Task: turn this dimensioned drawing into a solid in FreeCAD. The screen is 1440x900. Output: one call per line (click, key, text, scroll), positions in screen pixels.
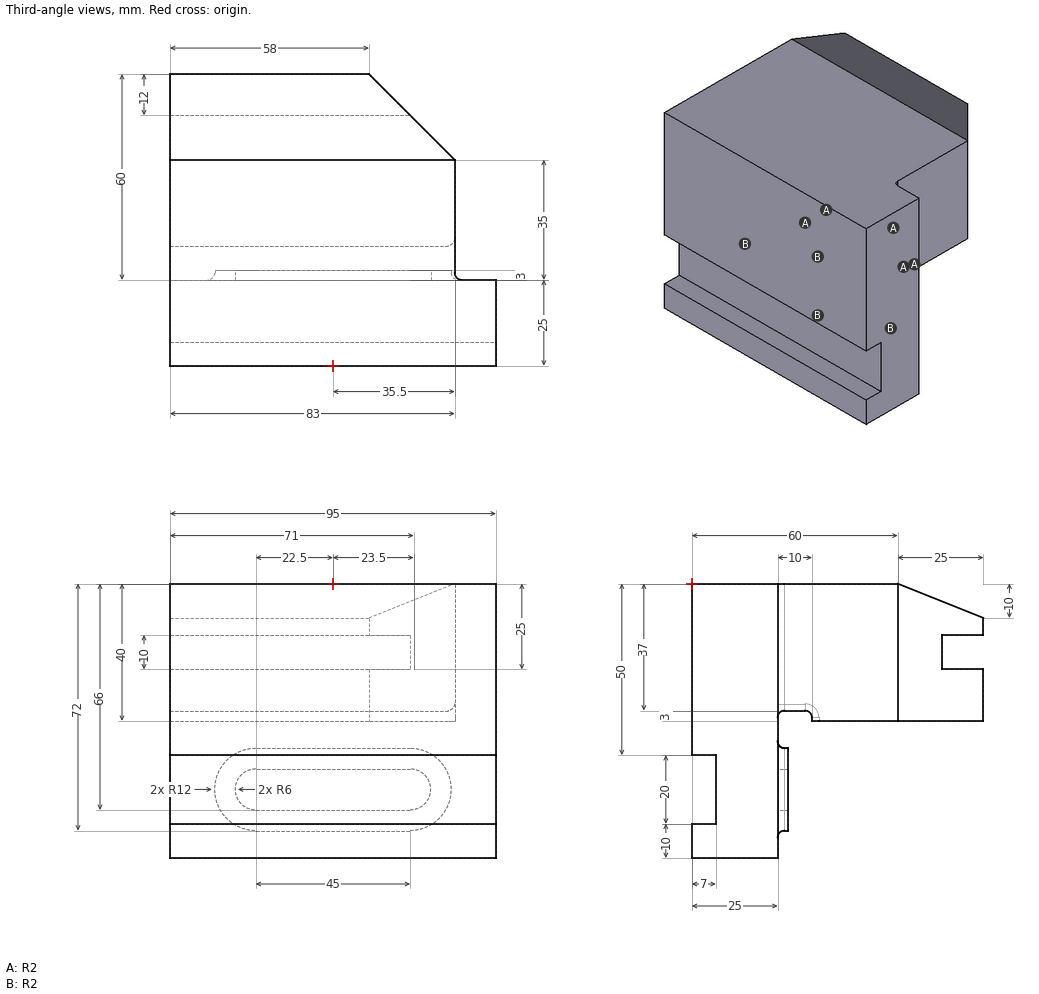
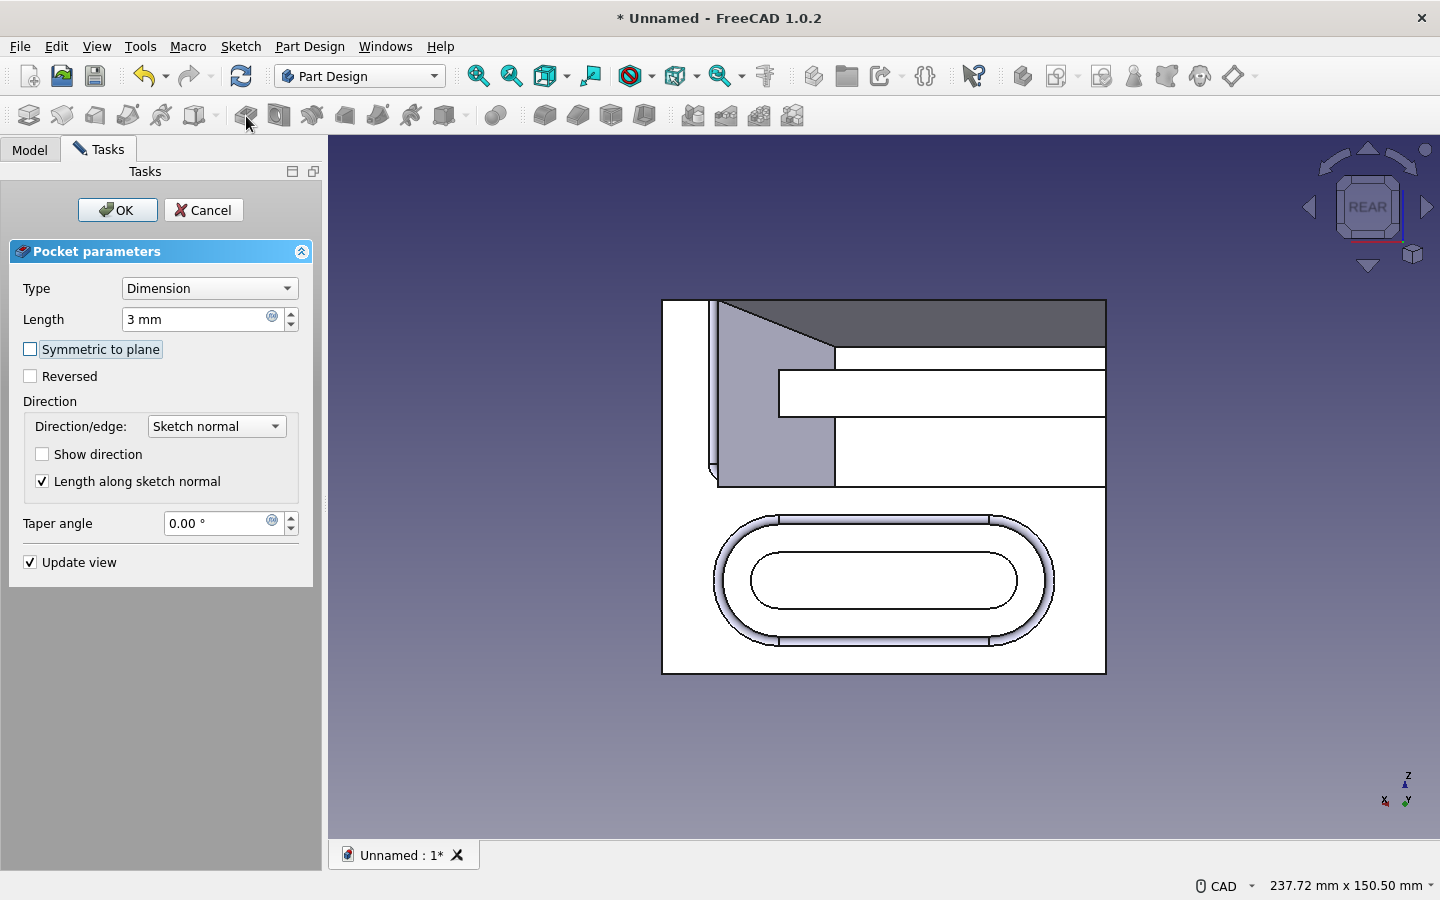
click(118, 210)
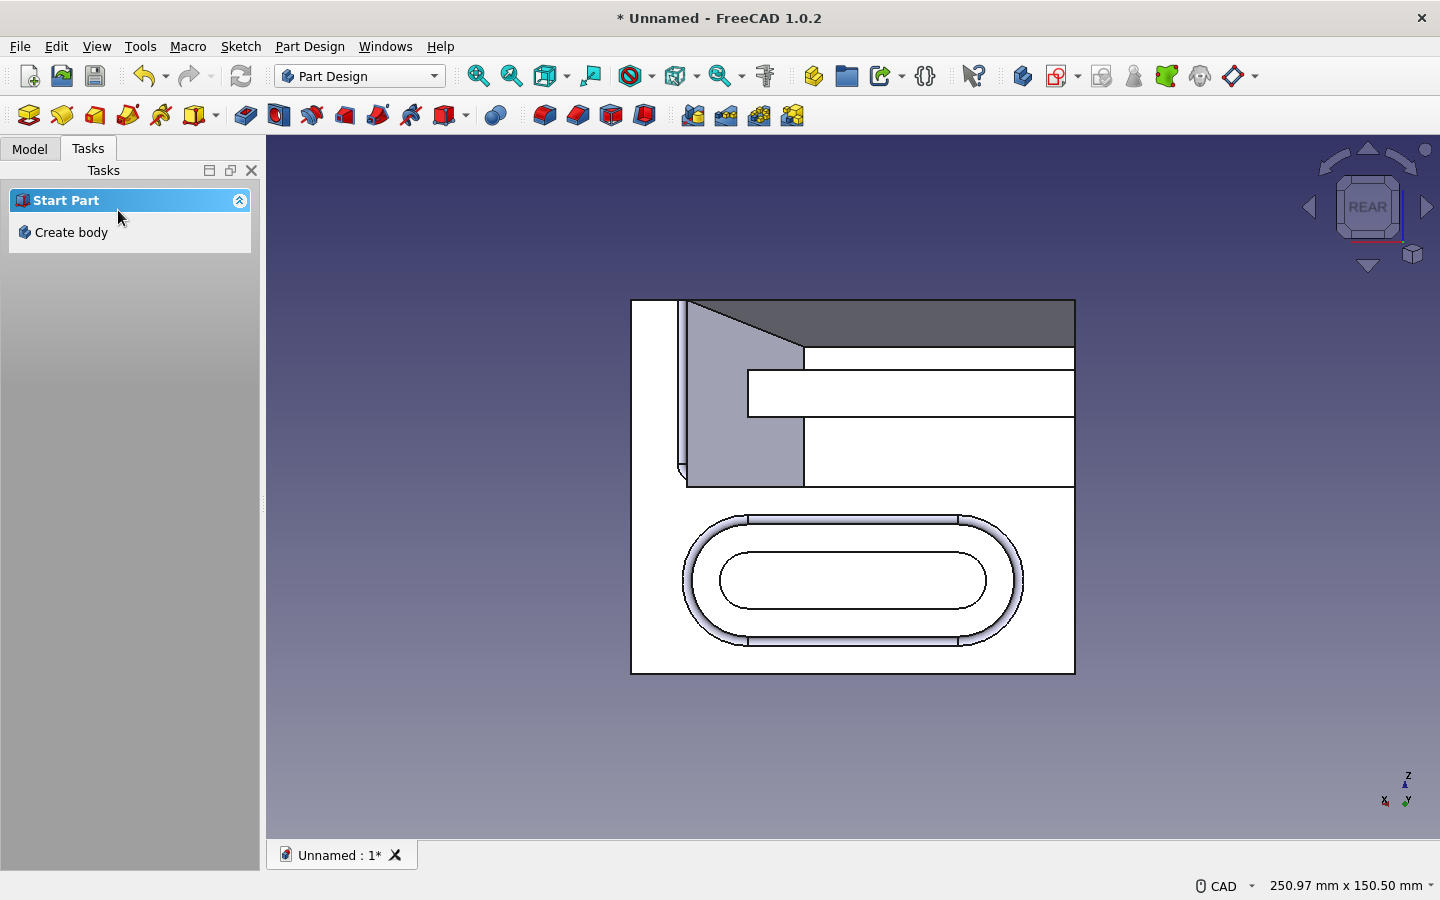
key(0)